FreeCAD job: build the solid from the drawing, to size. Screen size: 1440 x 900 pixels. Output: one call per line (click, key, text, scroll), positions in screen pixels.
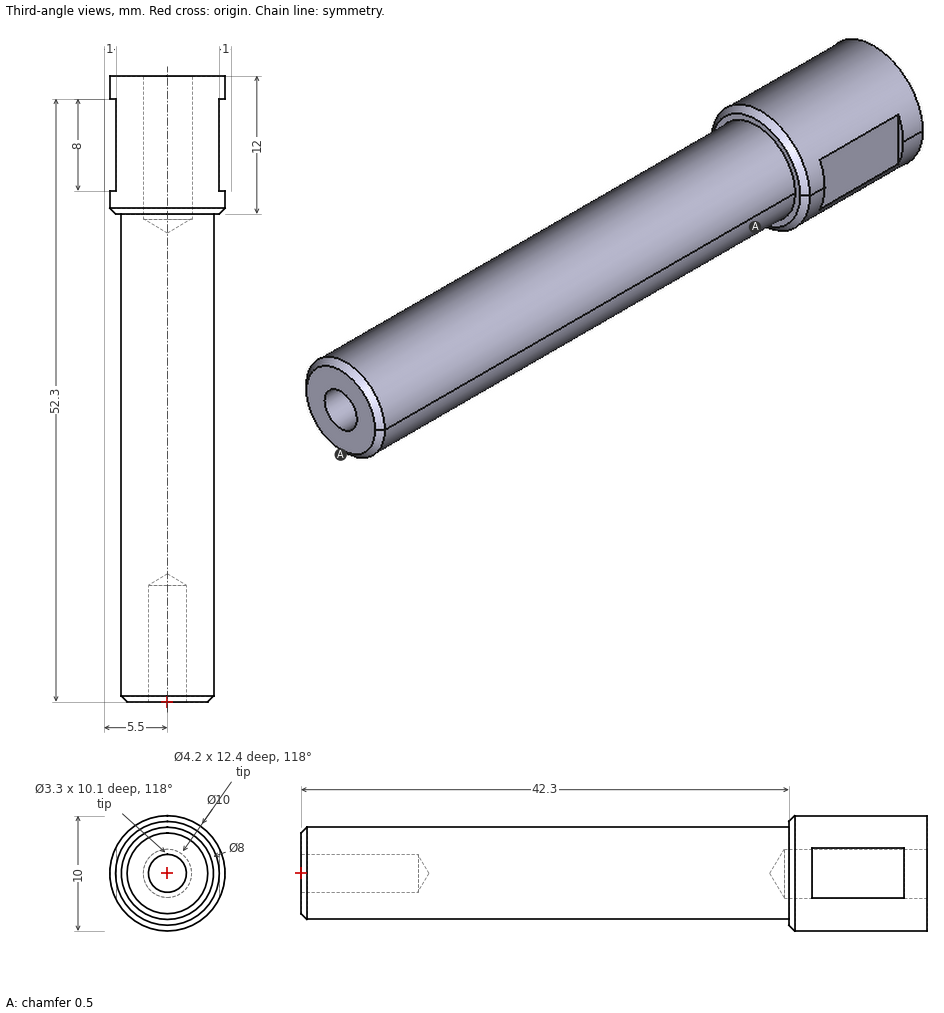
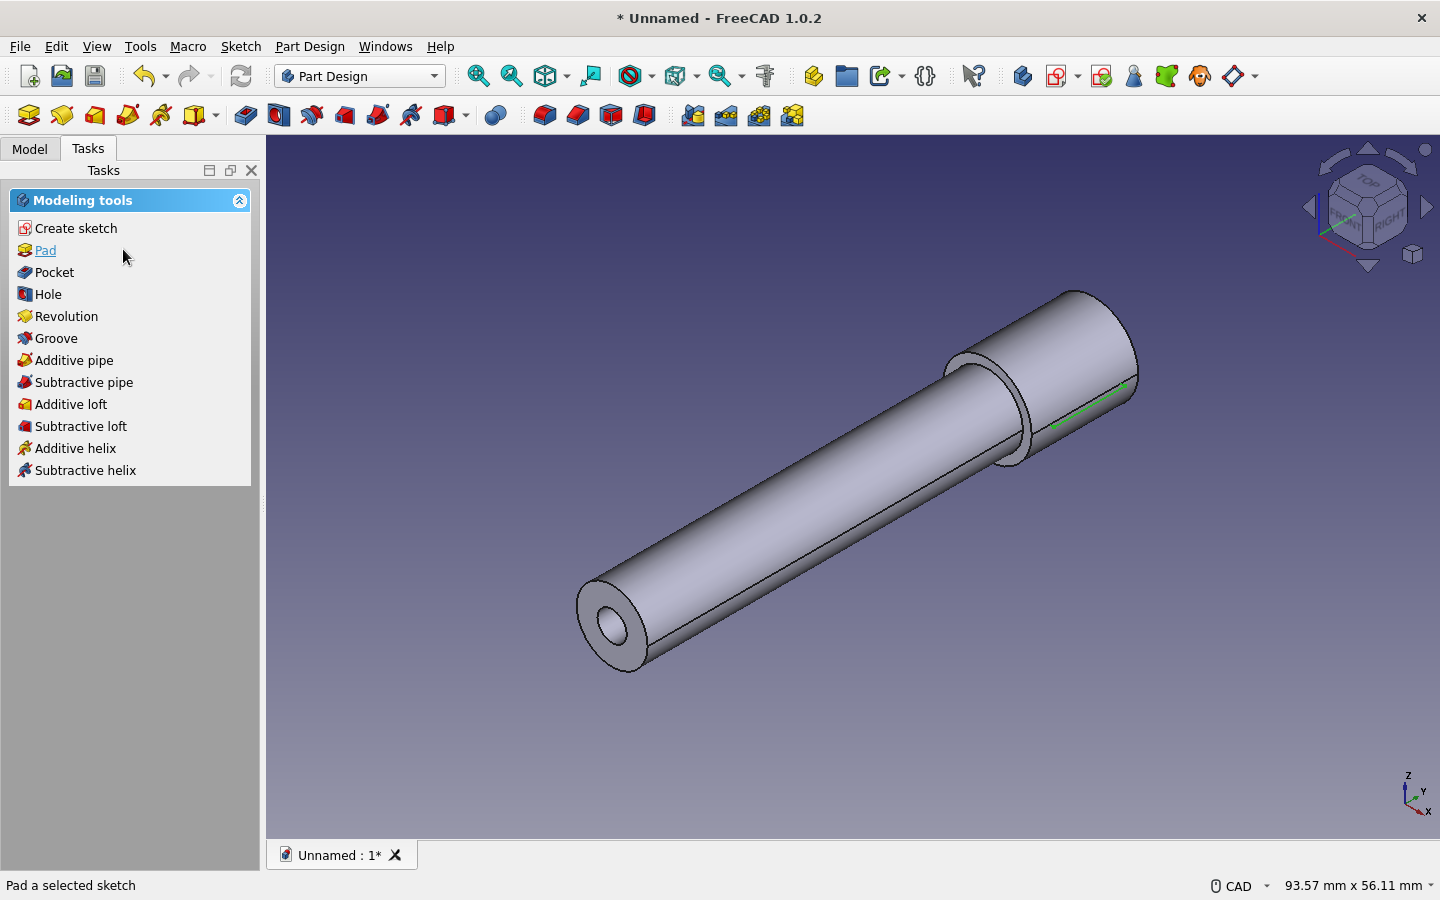
click(246, 116)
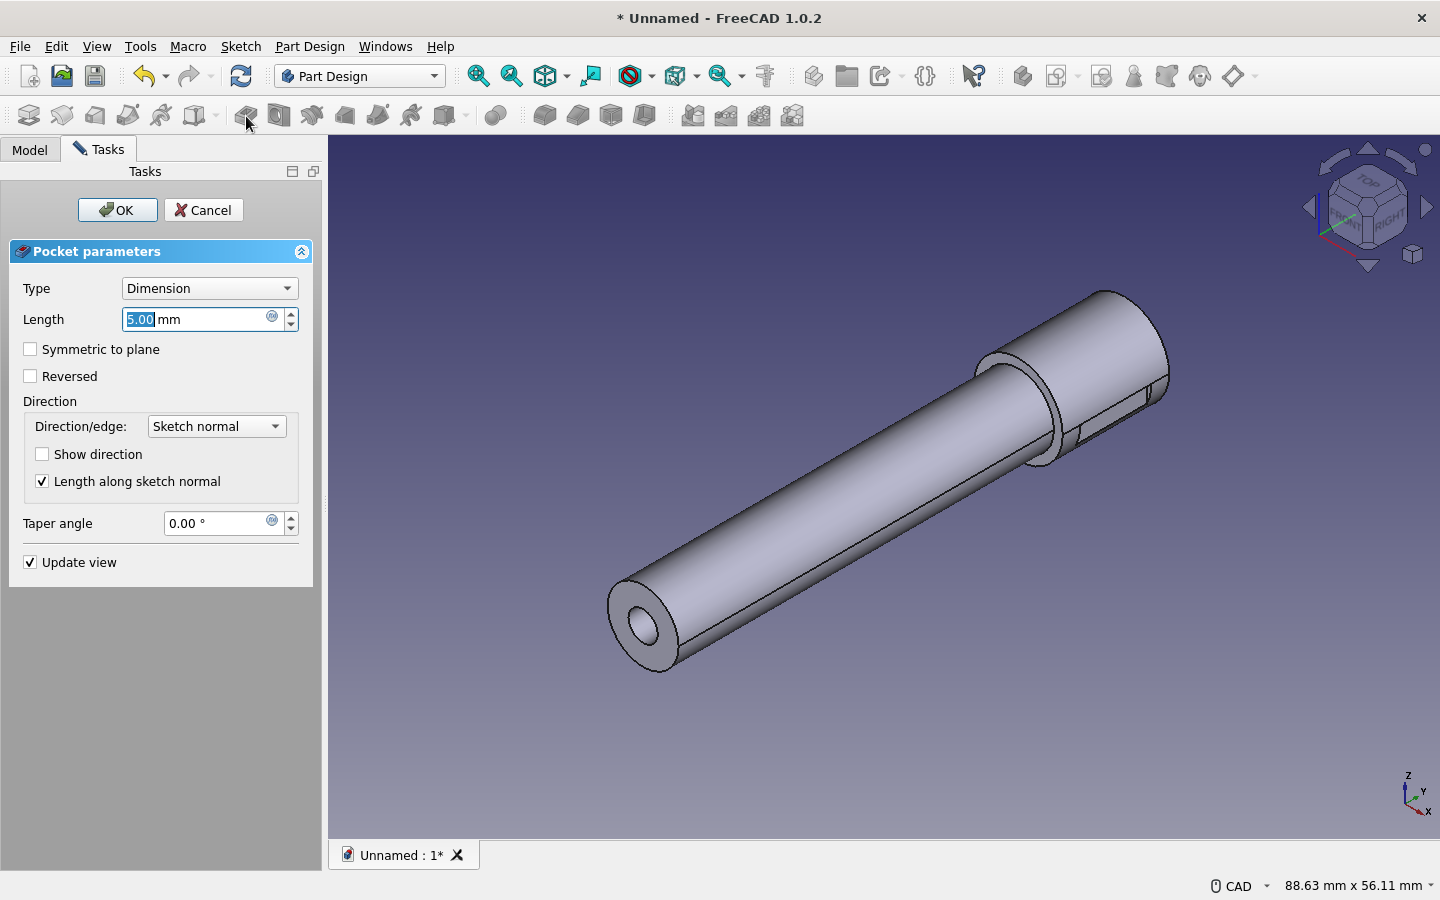
text(10)
key(Tab)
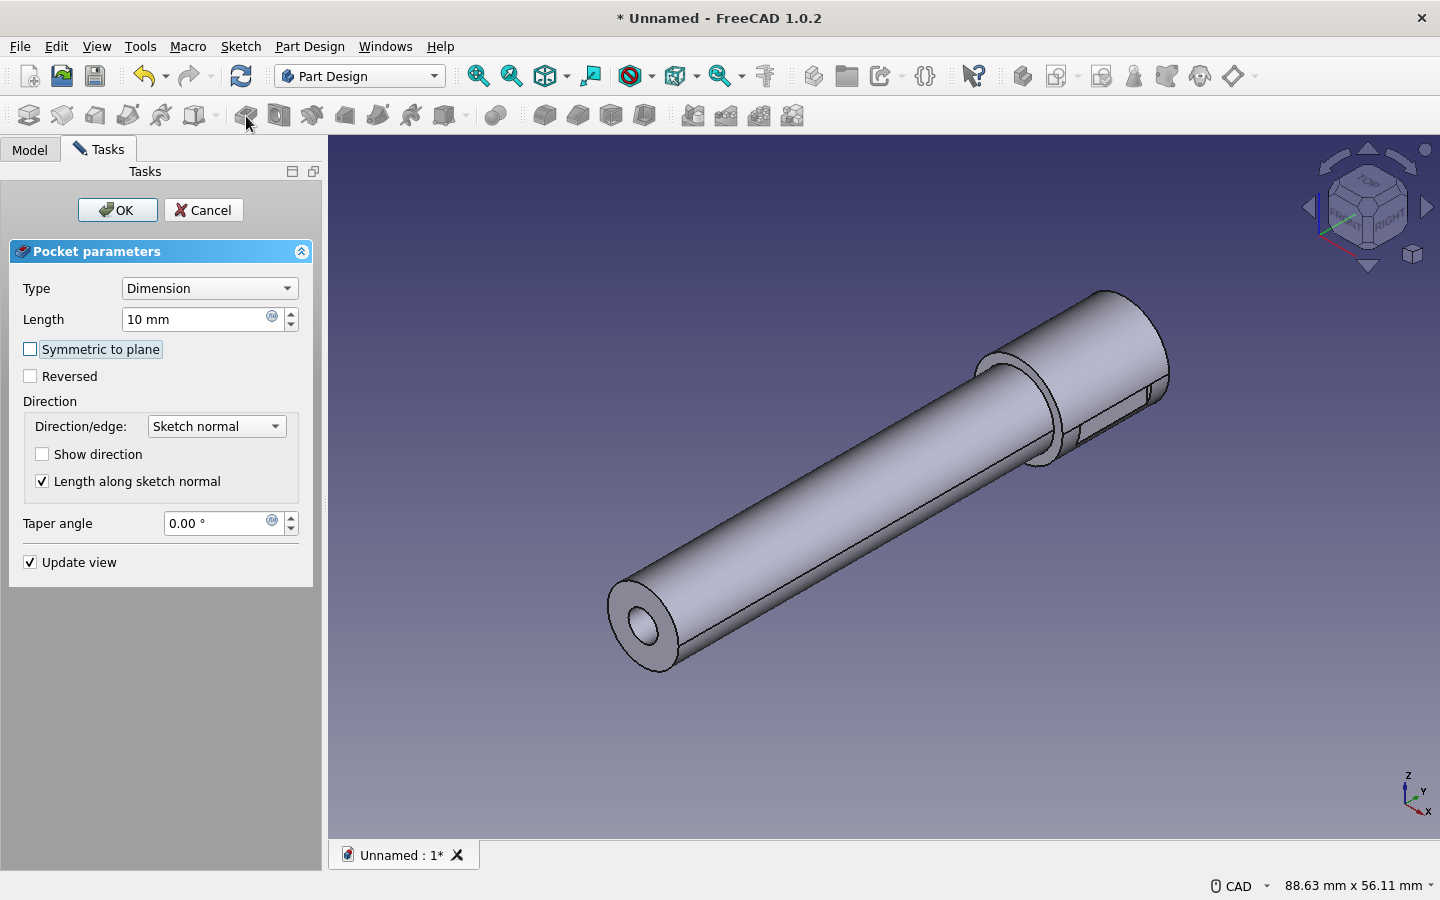
click(31, 349)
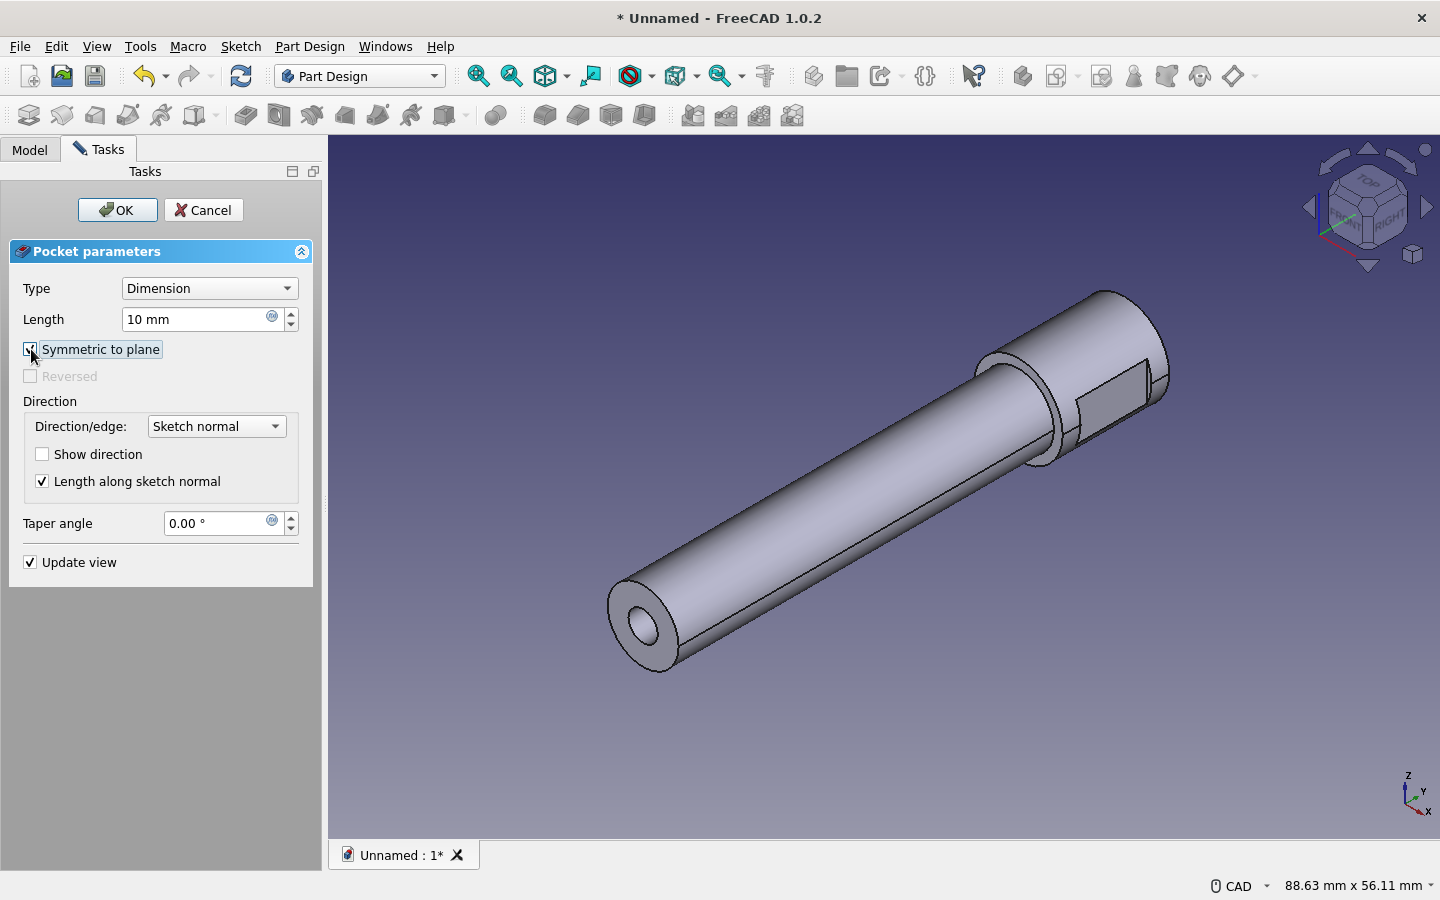
click(118, 210)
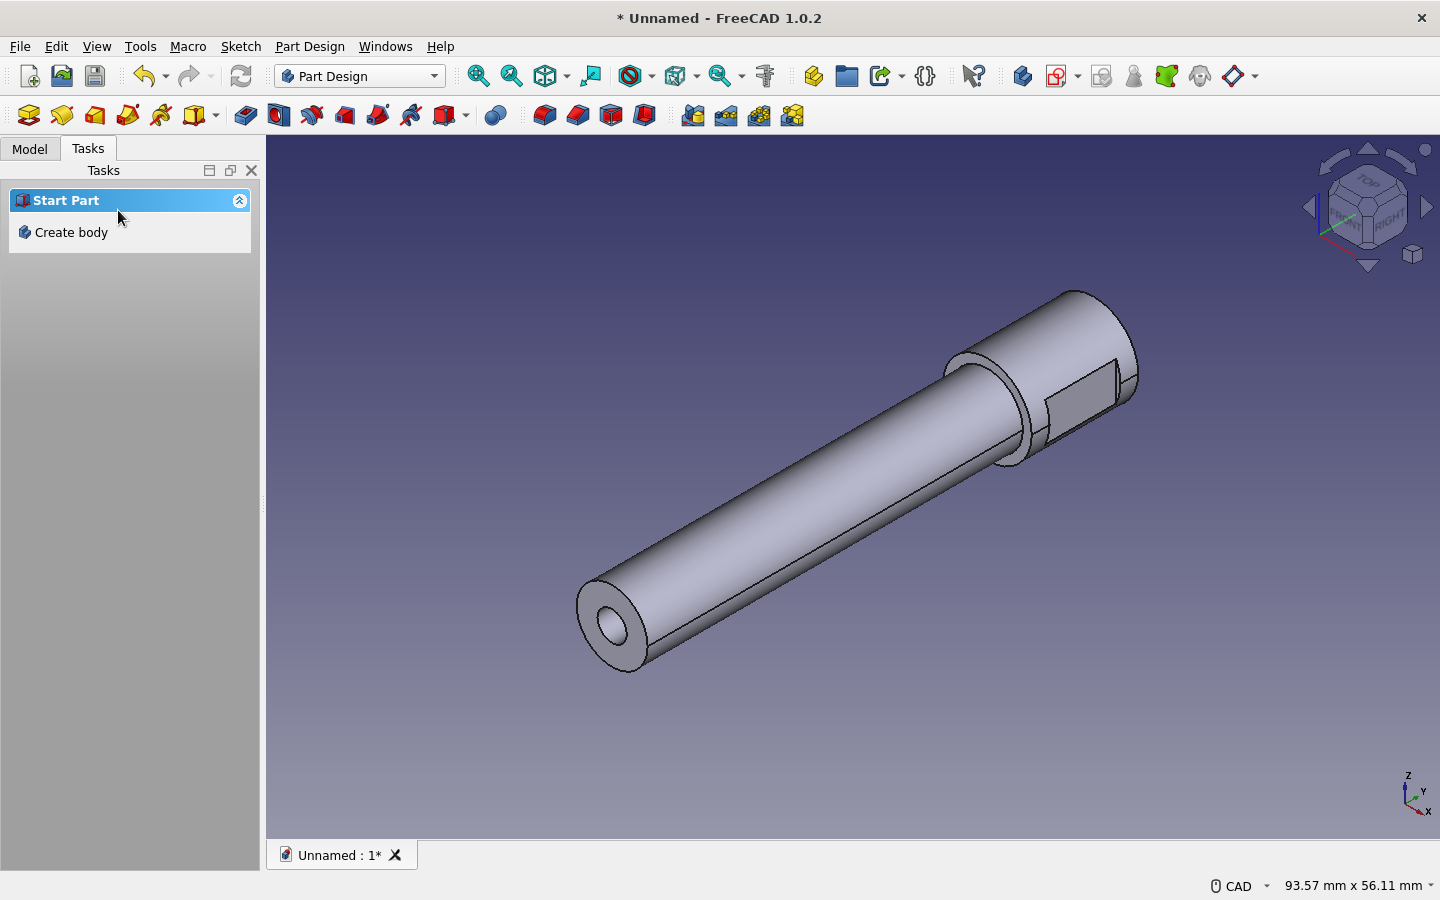
click(601, 580)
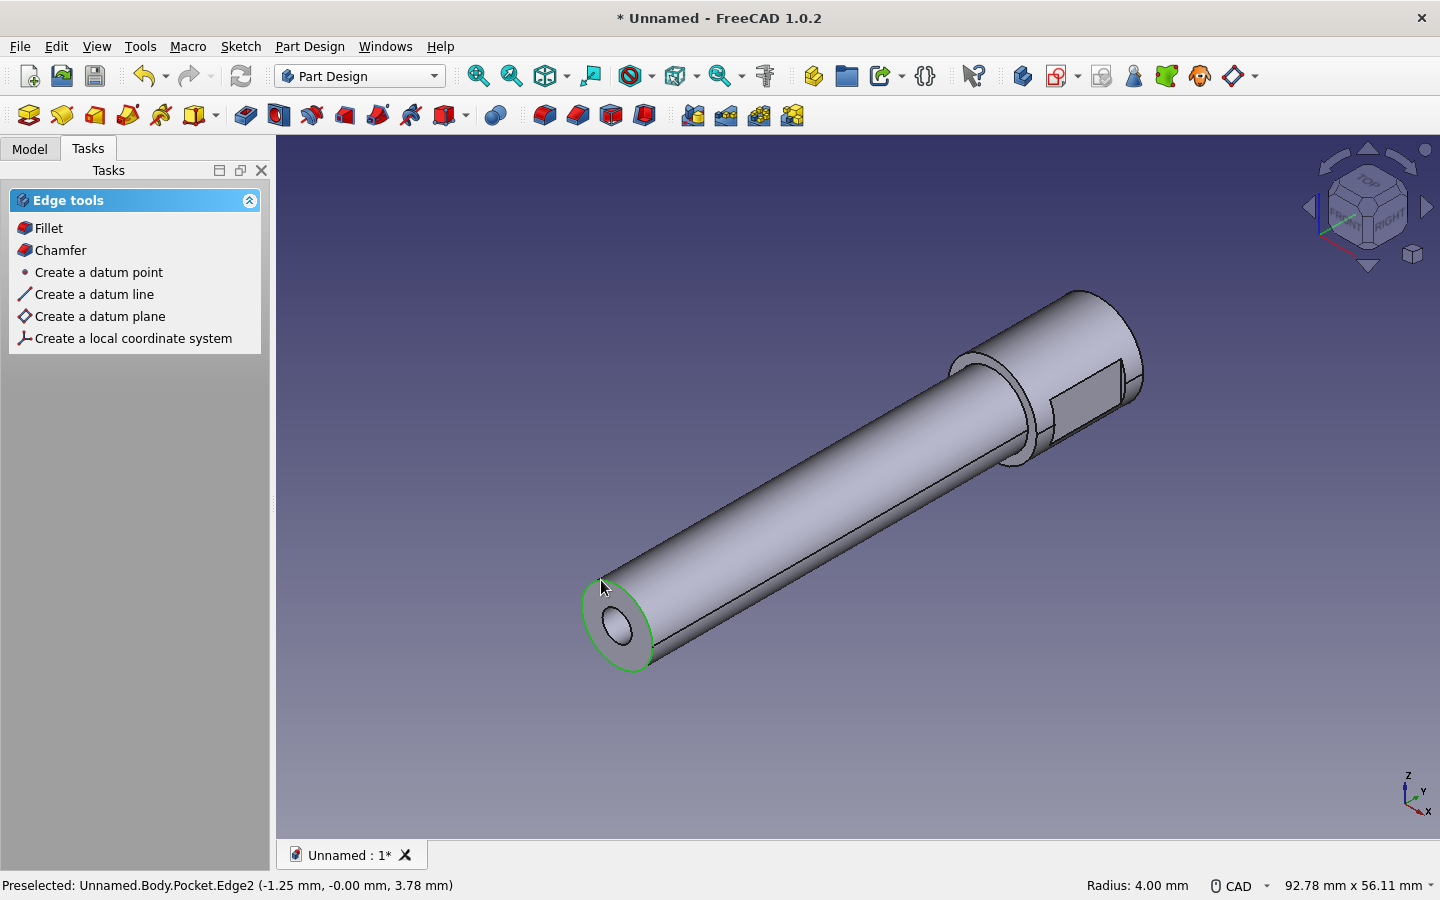
click(979, 352, ctrl)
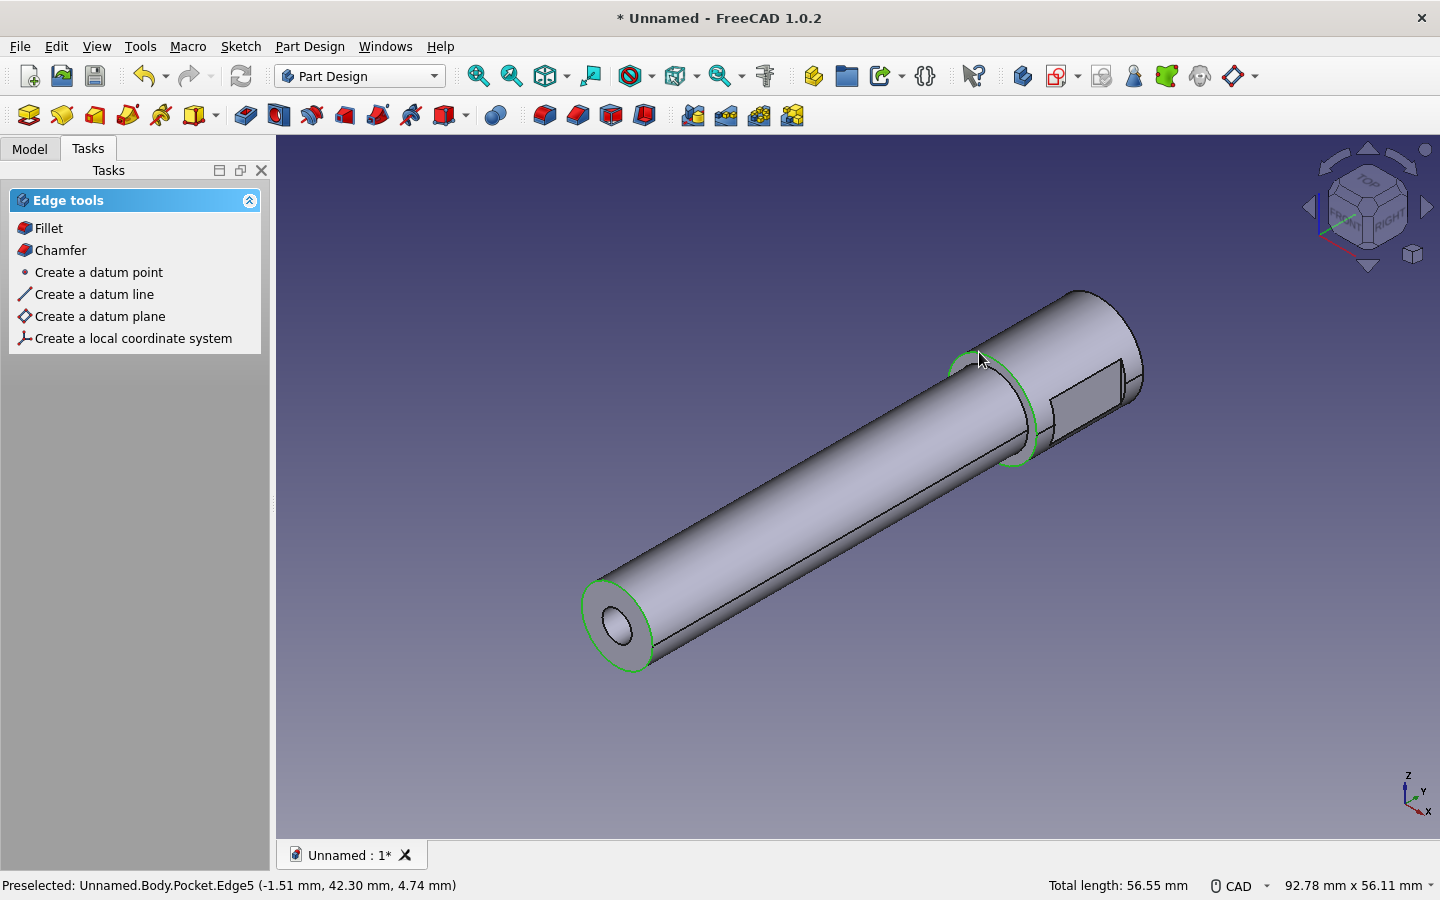
click(578, 116)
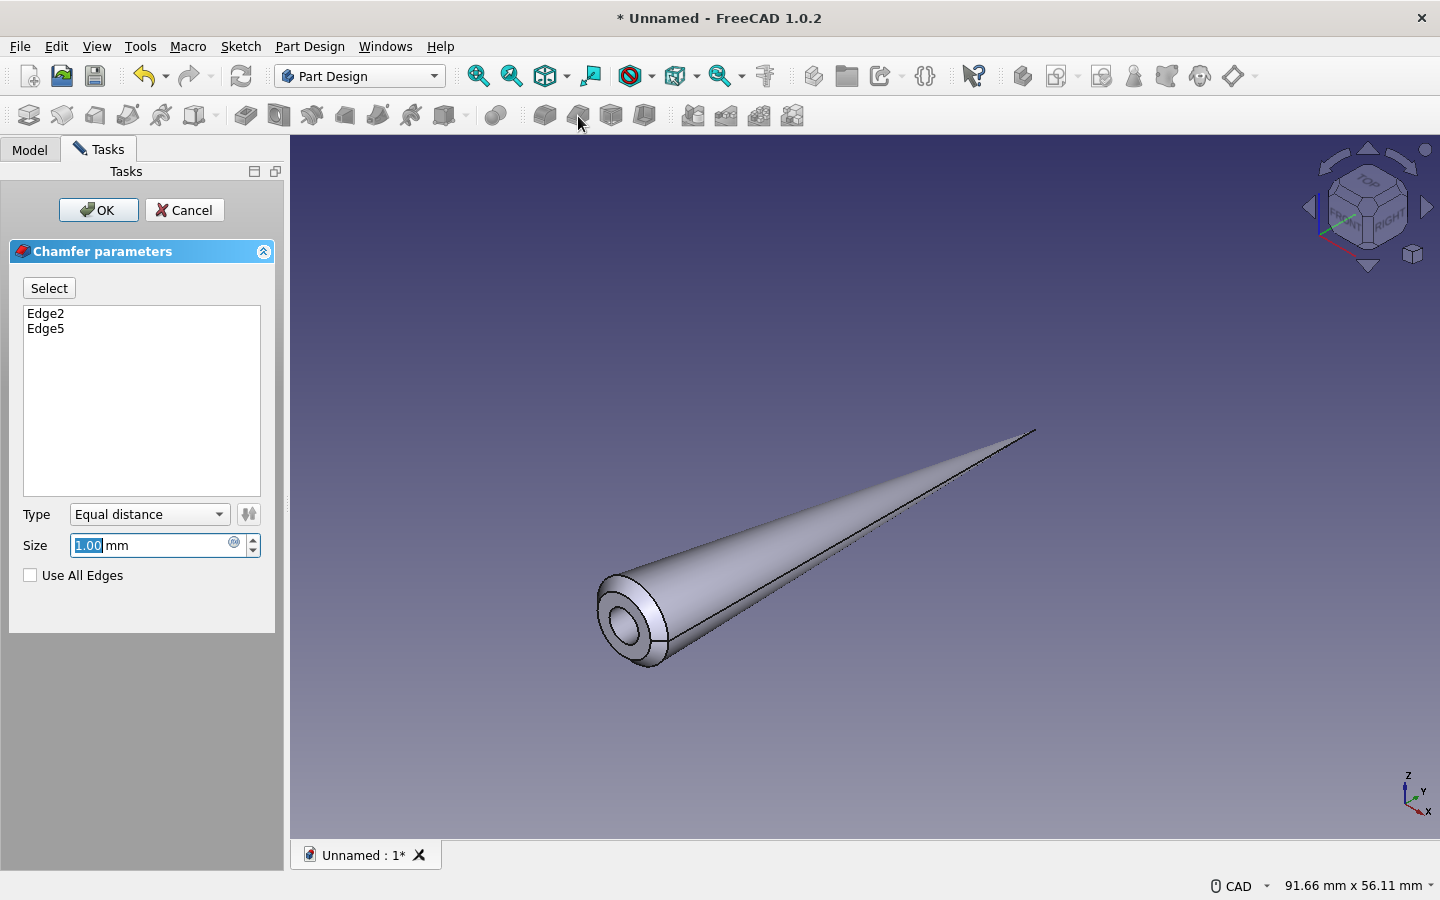
text(0.5)
key(Tab)